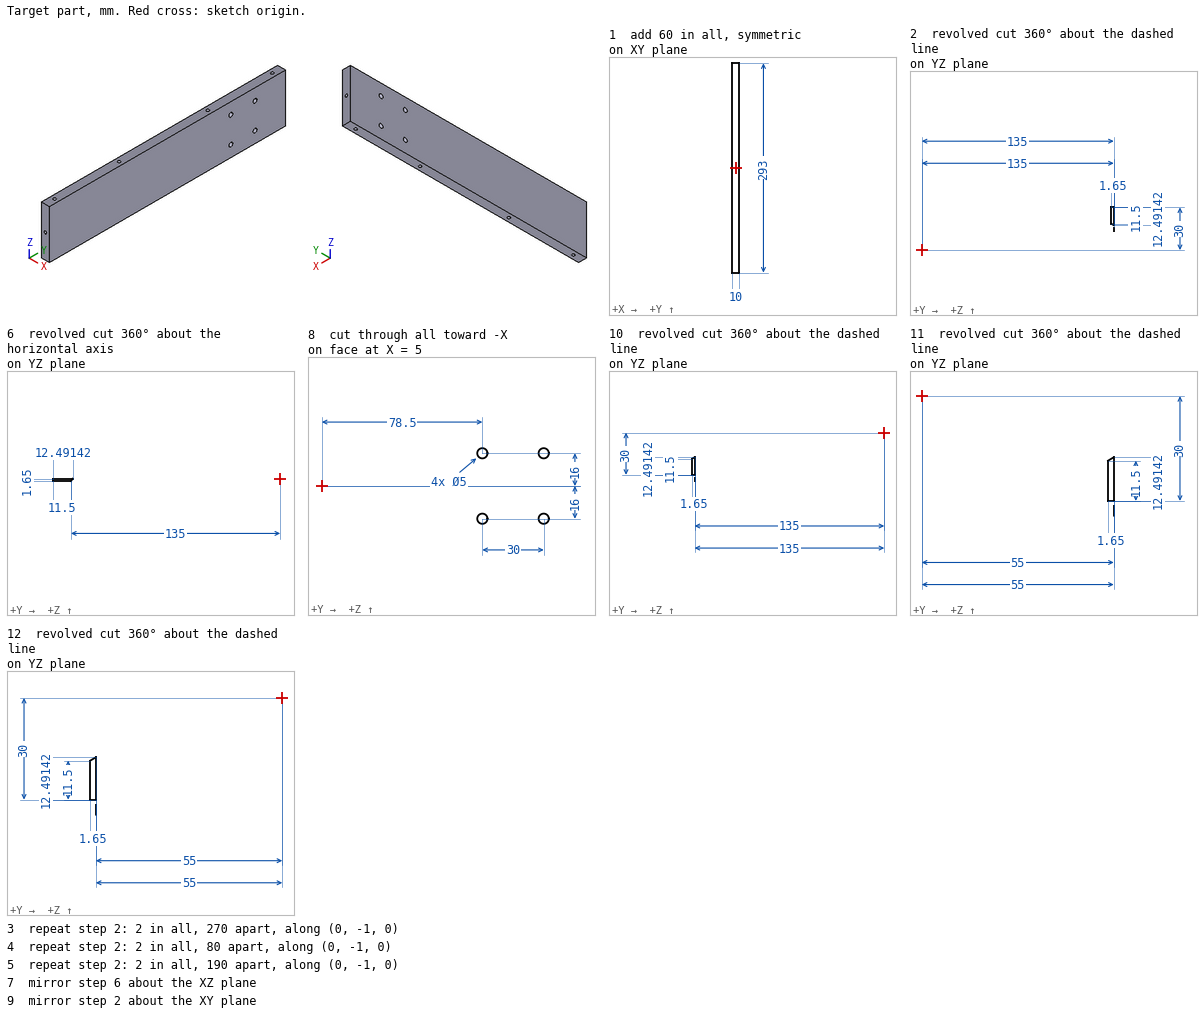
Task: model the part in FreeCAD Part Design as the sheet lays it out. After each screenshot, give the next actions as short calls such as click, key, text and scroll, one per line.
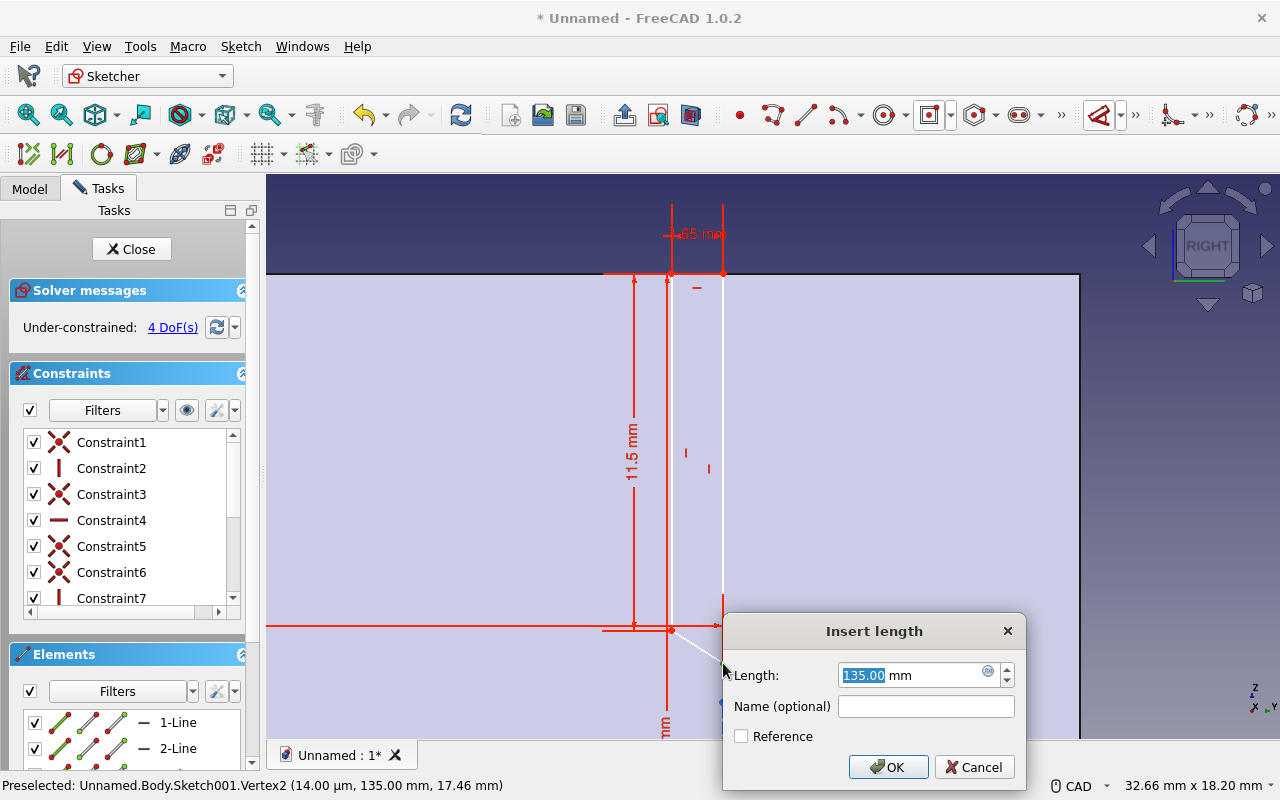
text(135)
key(Return)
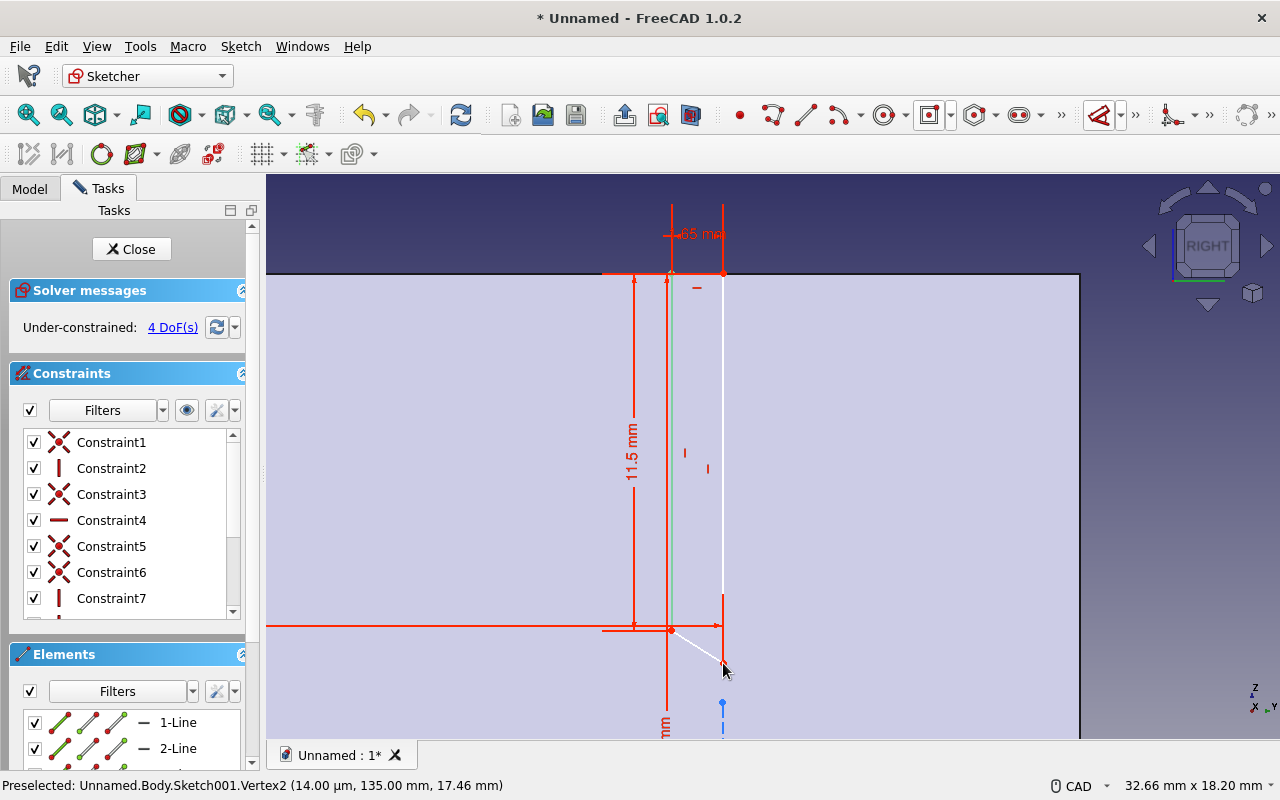
click(723, 702)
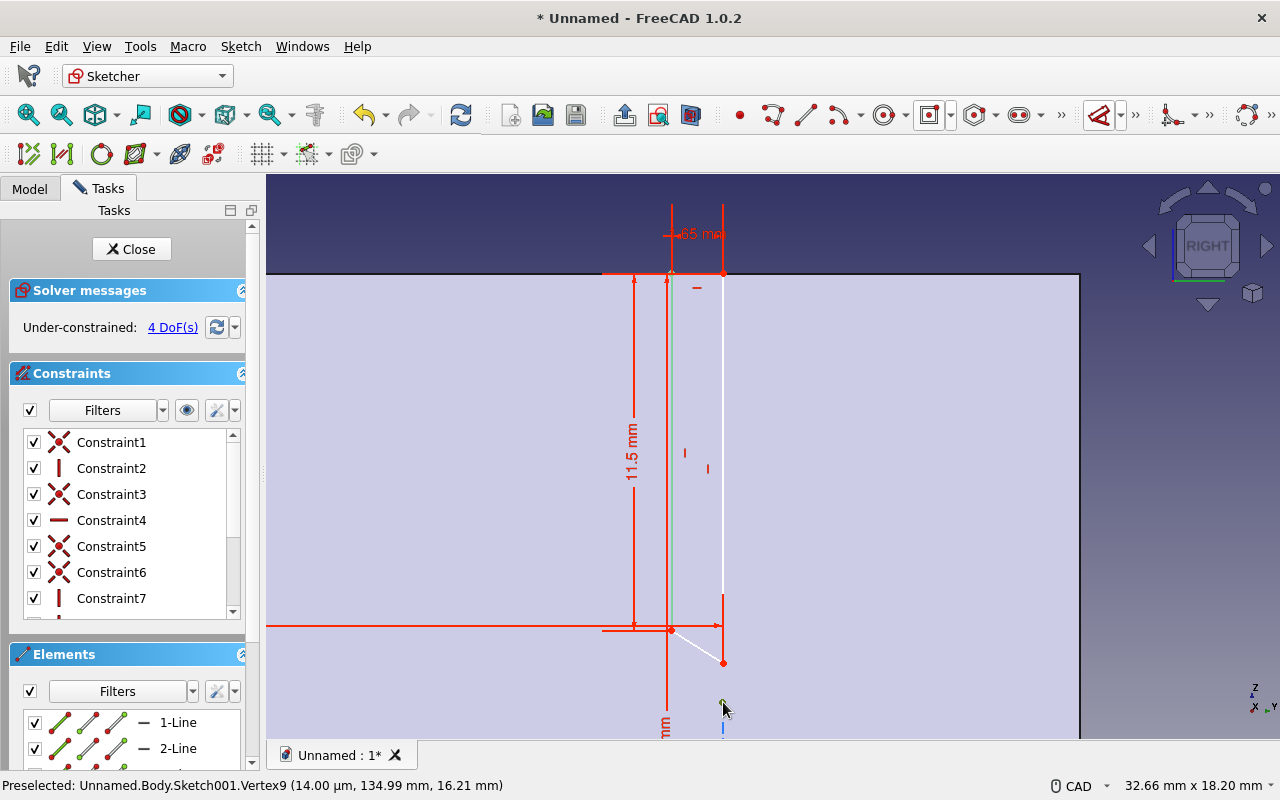
click(1120, 116)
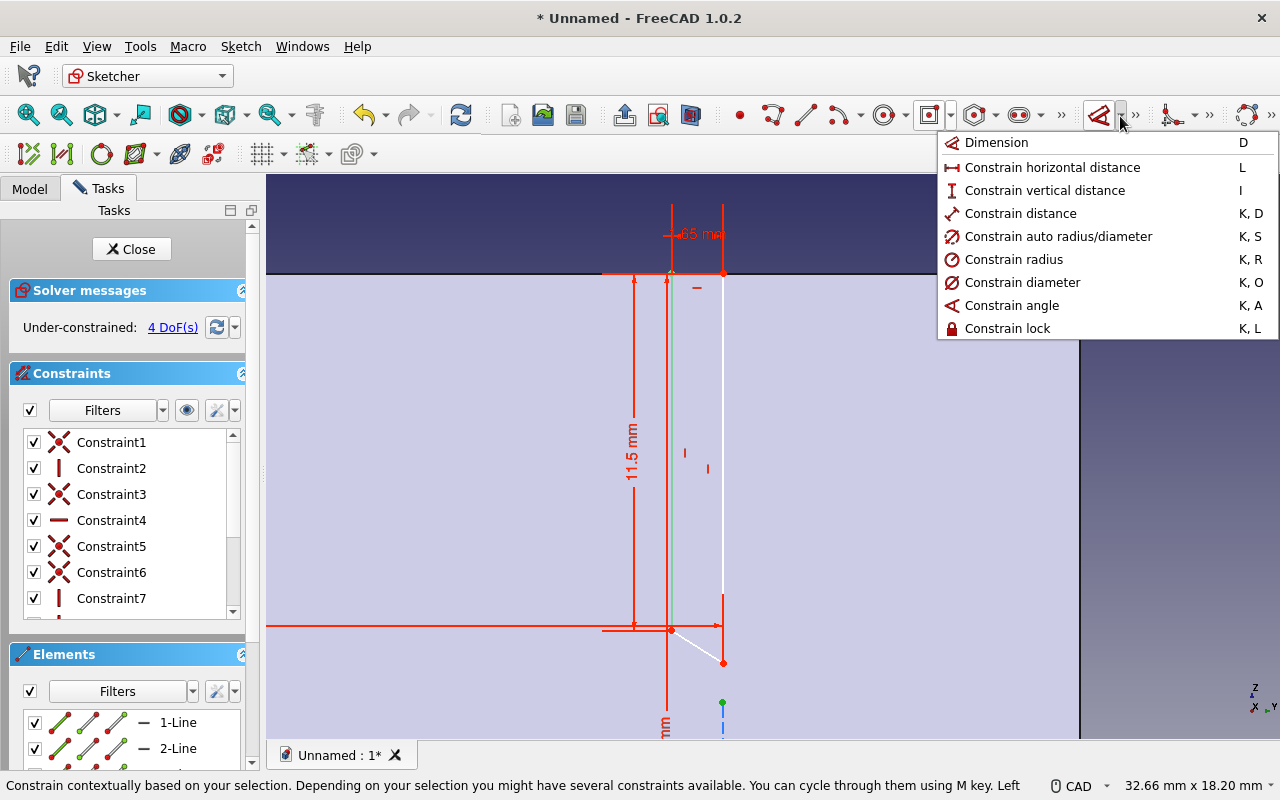
click(1108, 168)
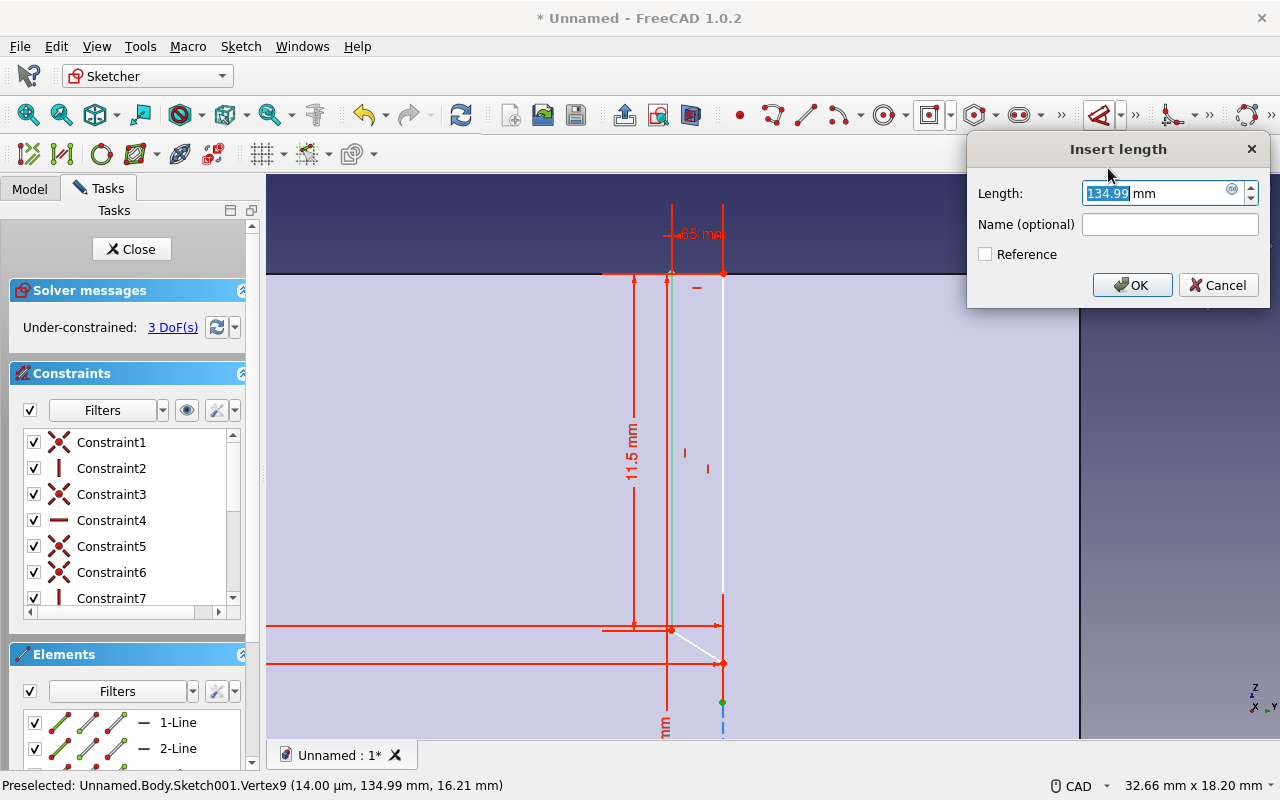
text(135)
key(Return)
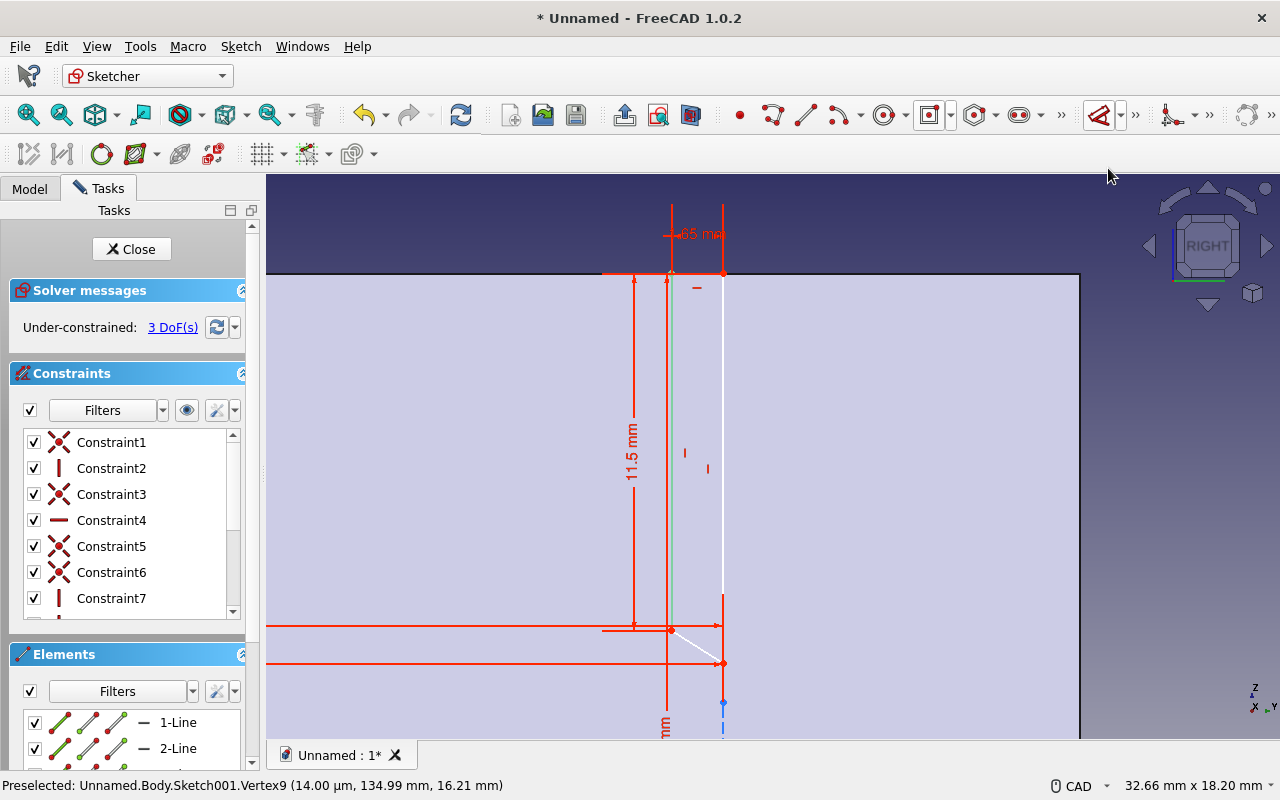
click(723, 546)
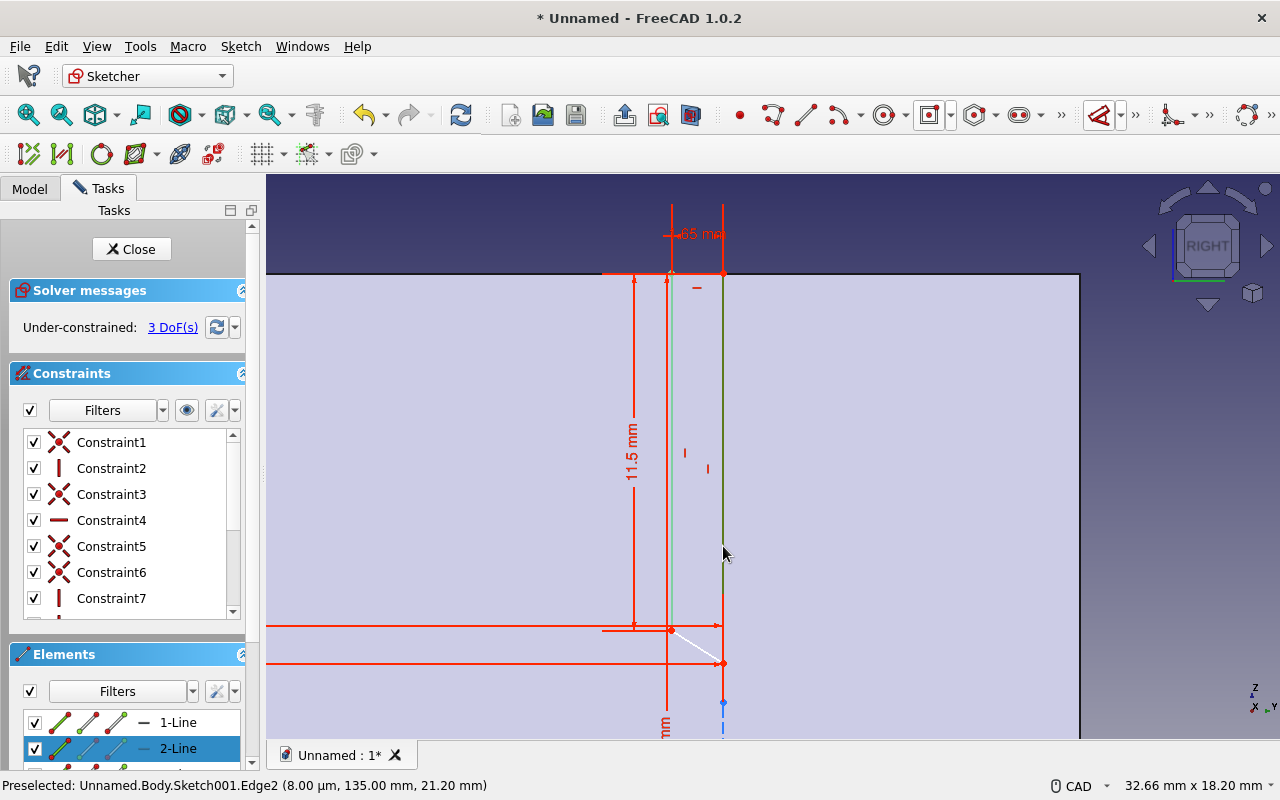
click(1120, 116)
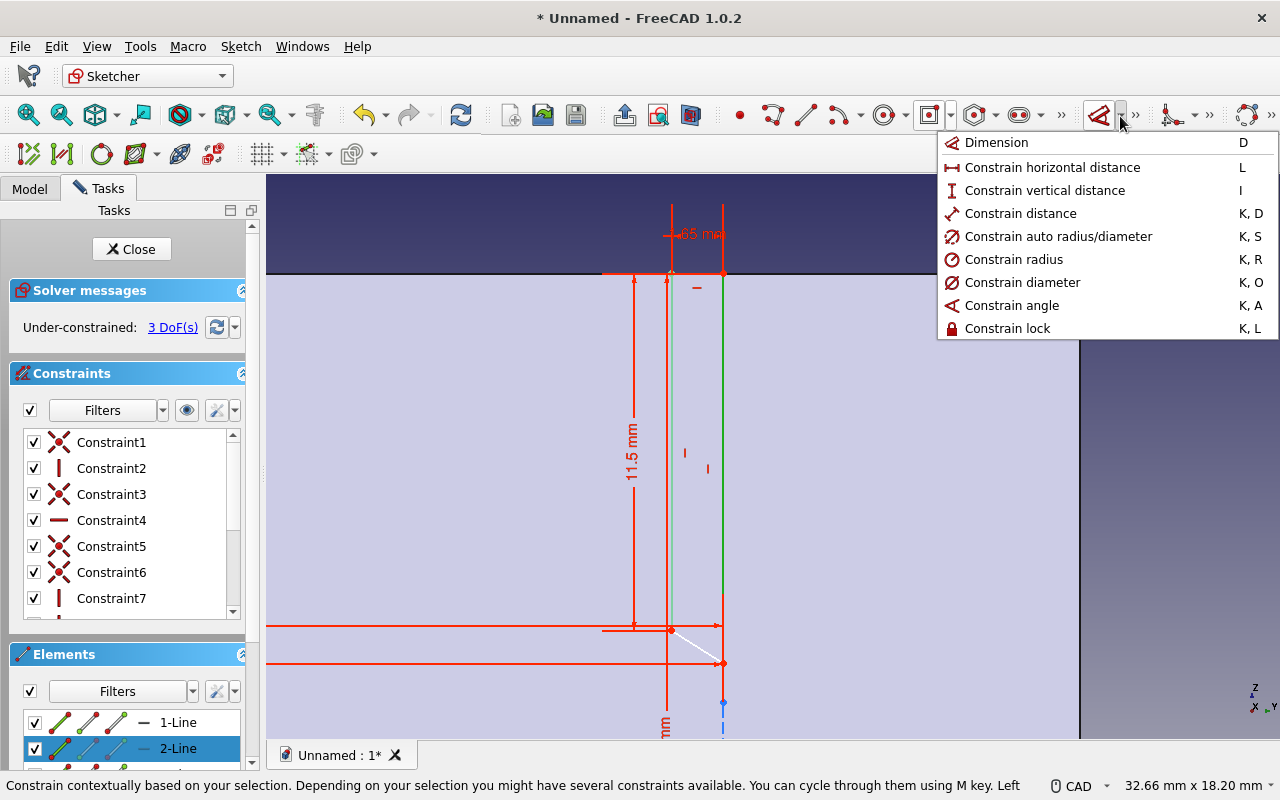
click(1108, 190)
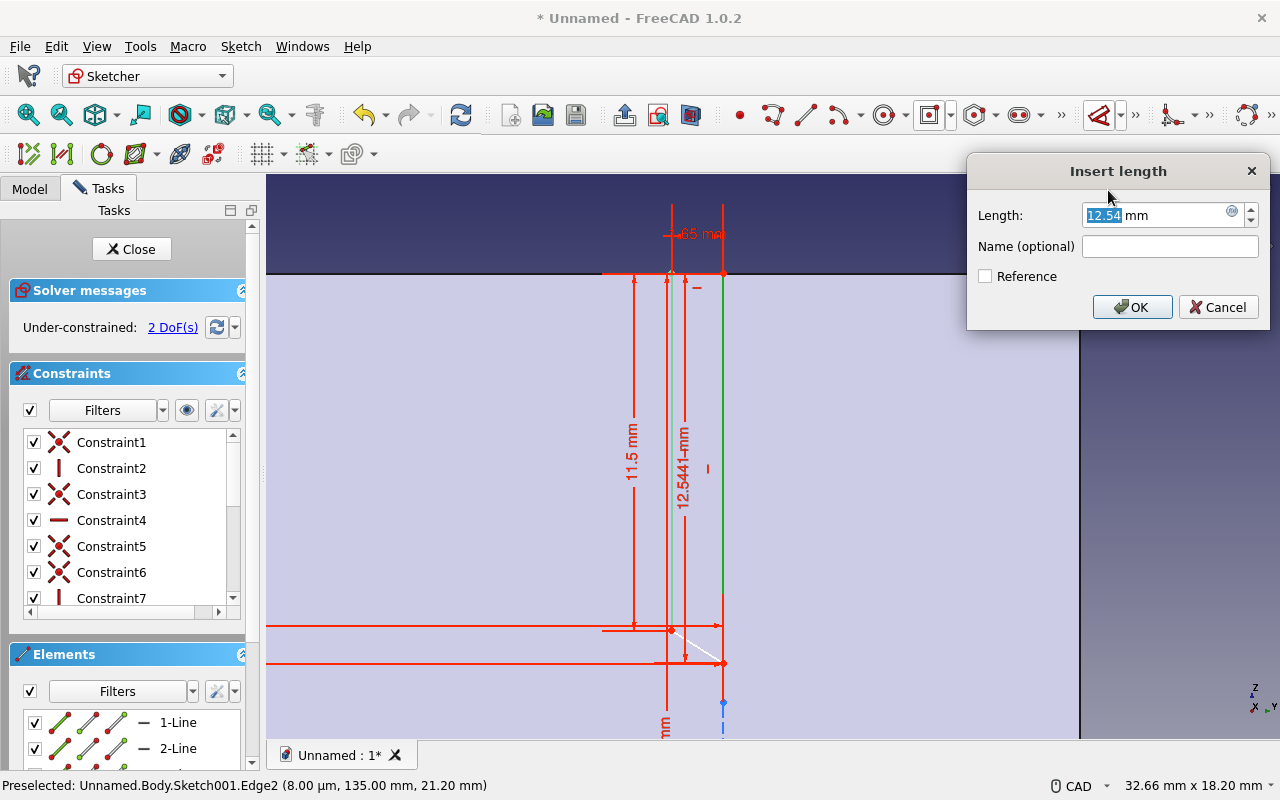
text(12.49142)
key(Return)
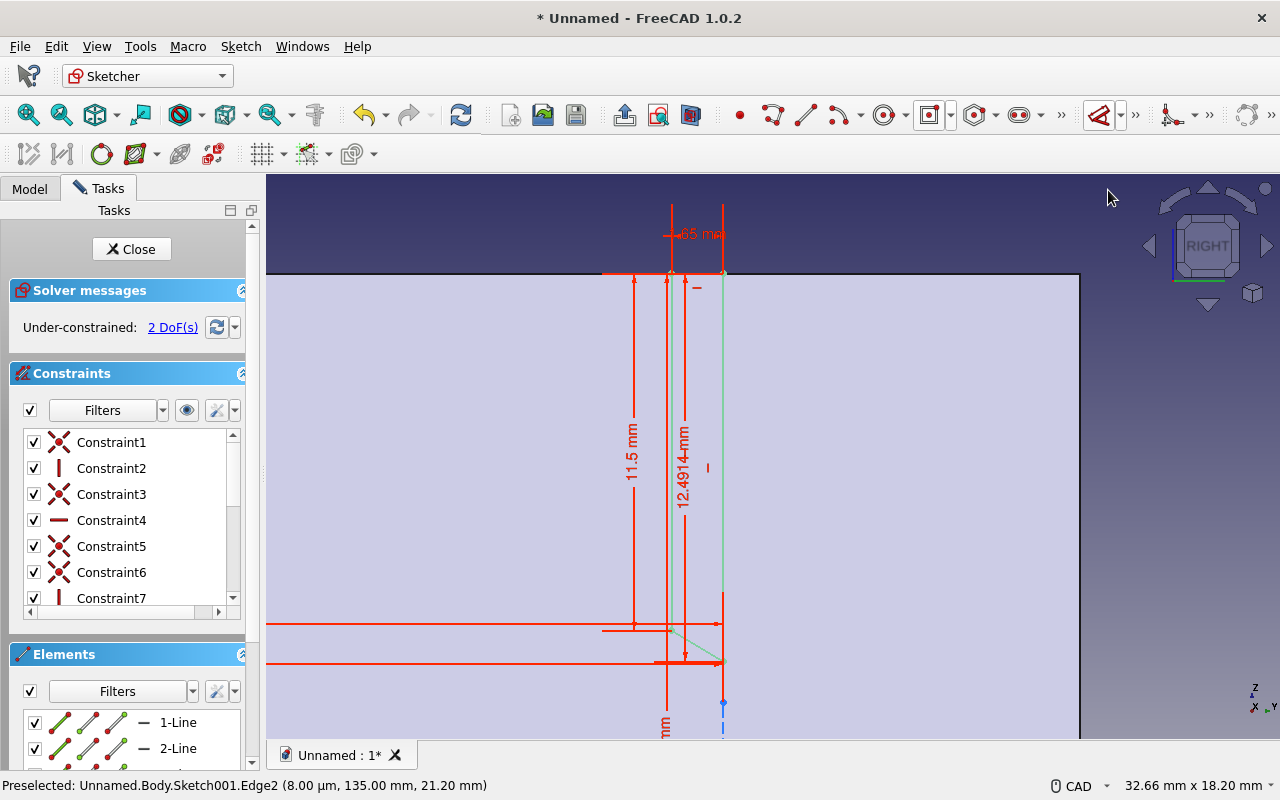
click(132, 249)